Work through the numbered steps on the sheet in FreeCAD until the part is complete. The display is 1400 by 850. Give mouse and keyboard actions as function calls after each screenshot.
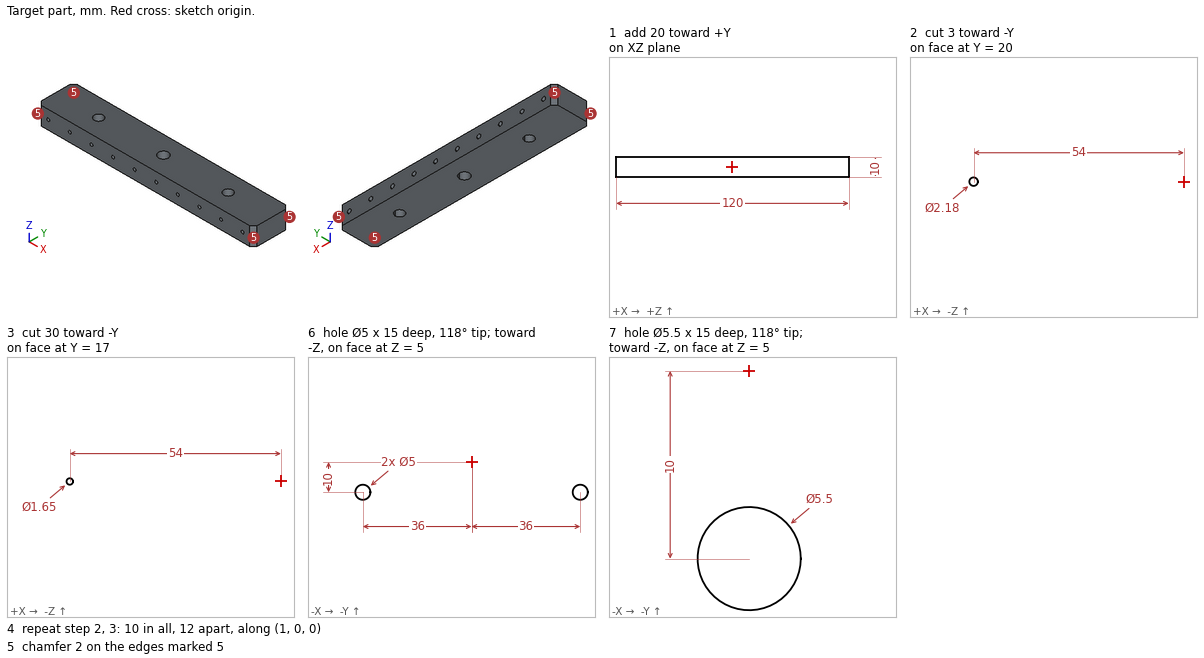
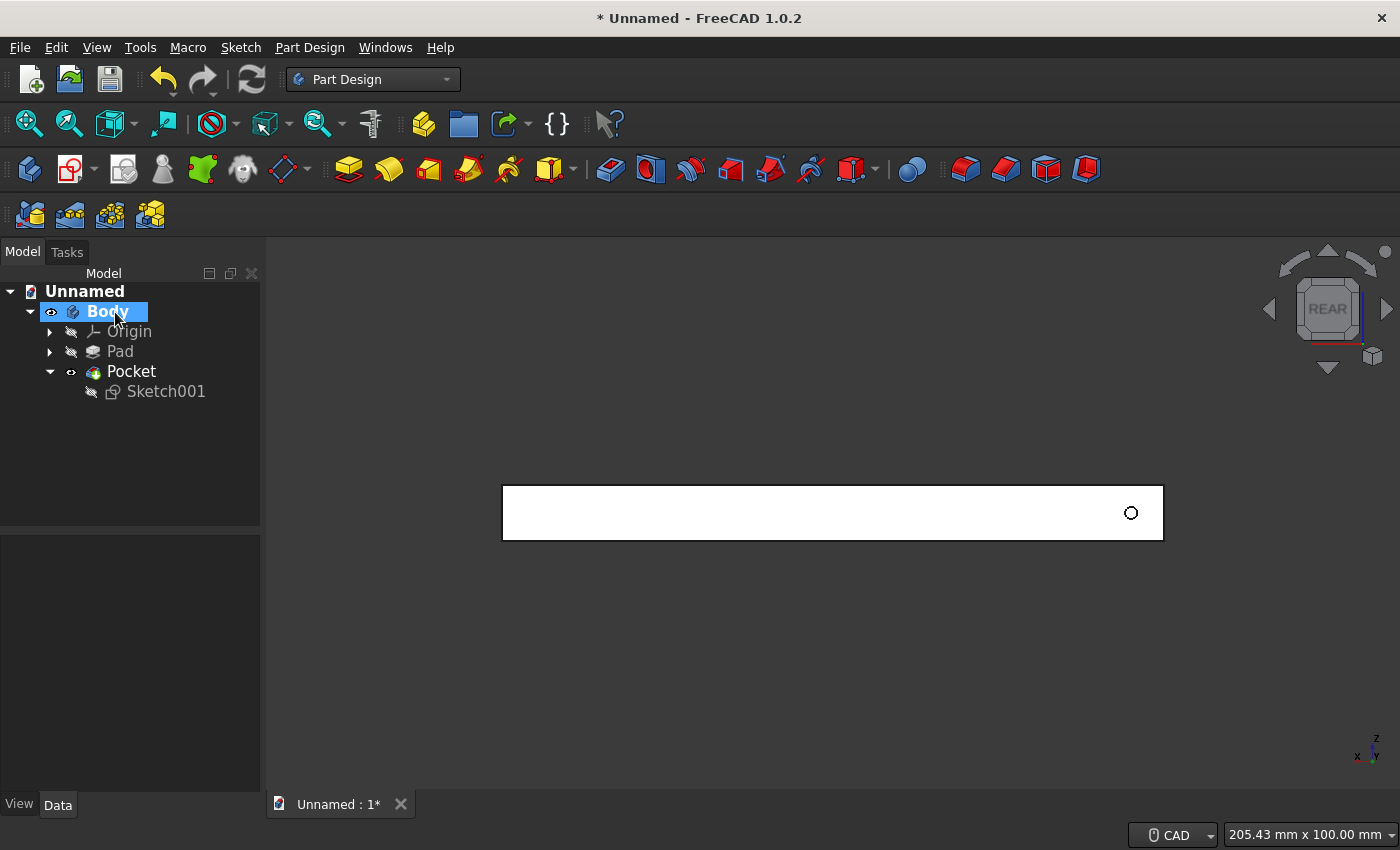
scroll(1131, 512, up, 4)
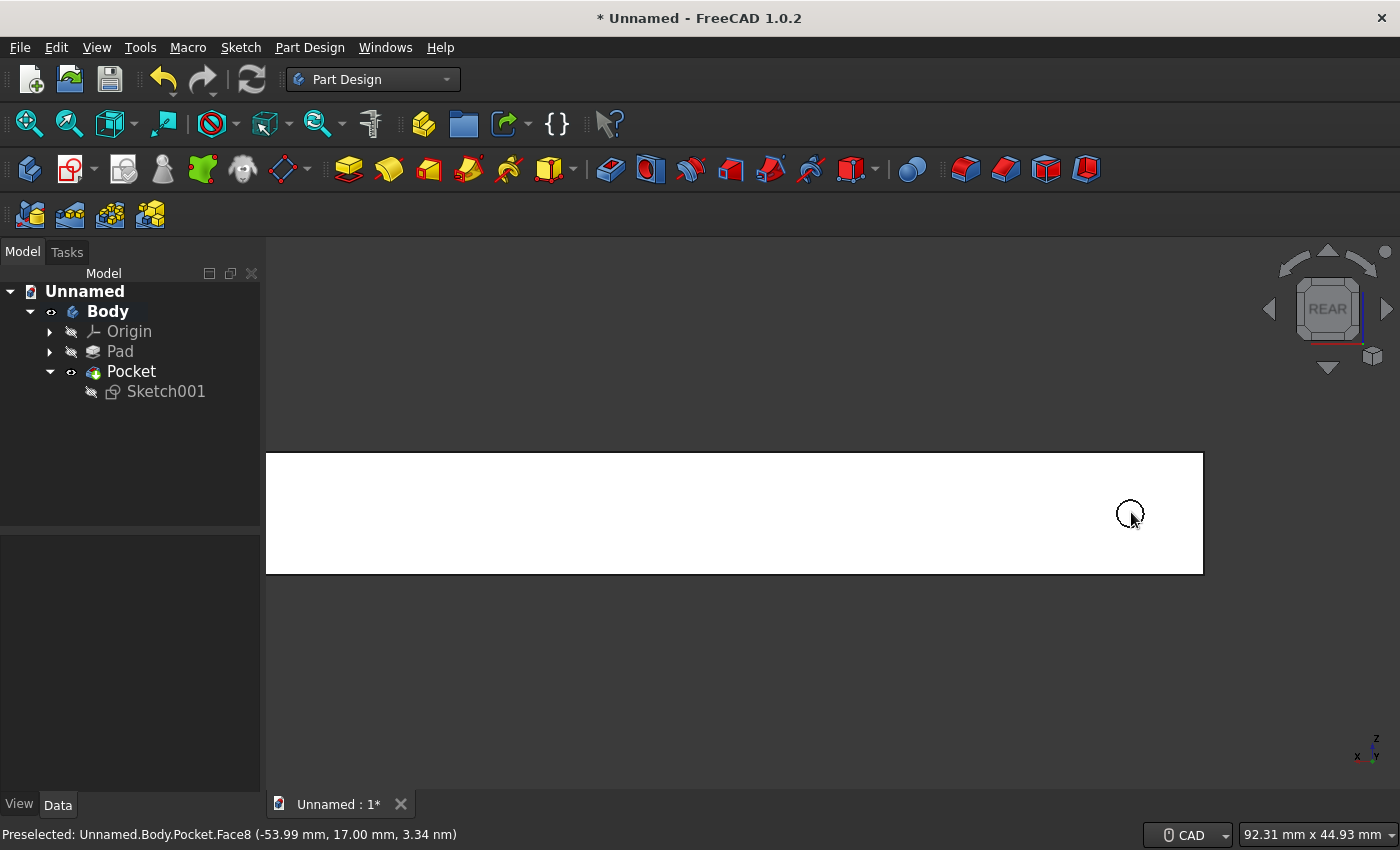
click(1130, 513)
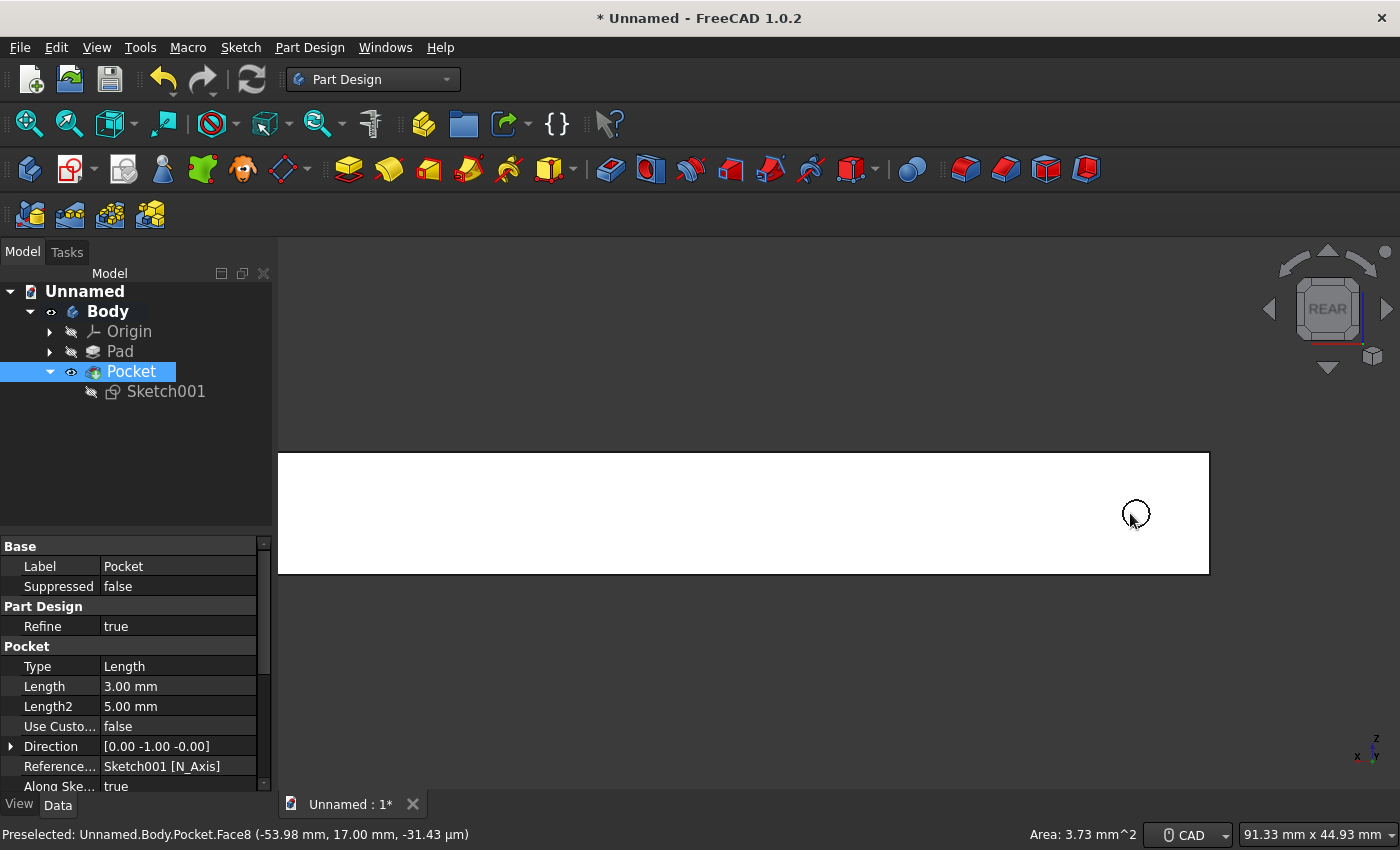
click(70, 170)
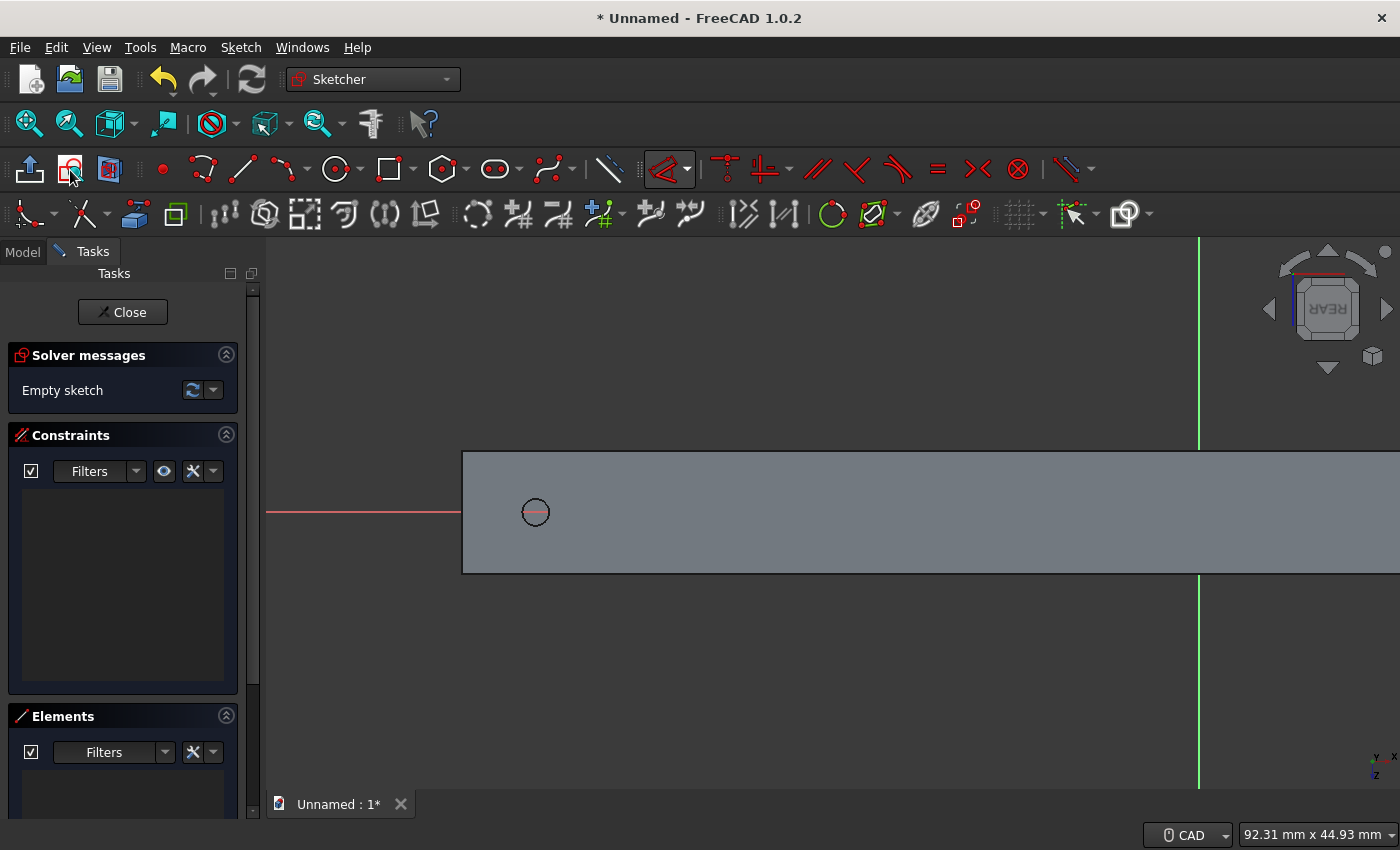
scroll(521, 512, up, 14)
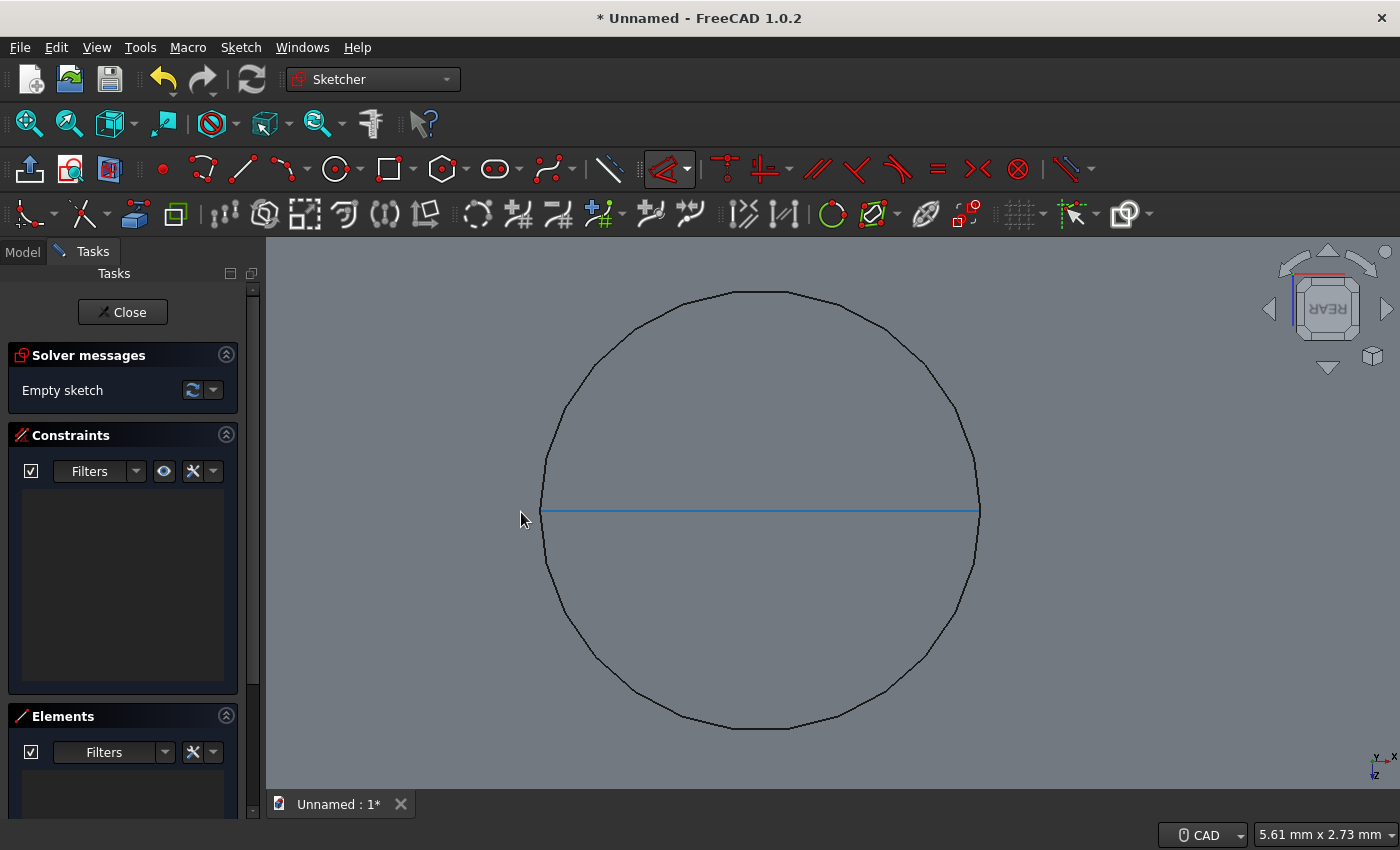
click(336, 170)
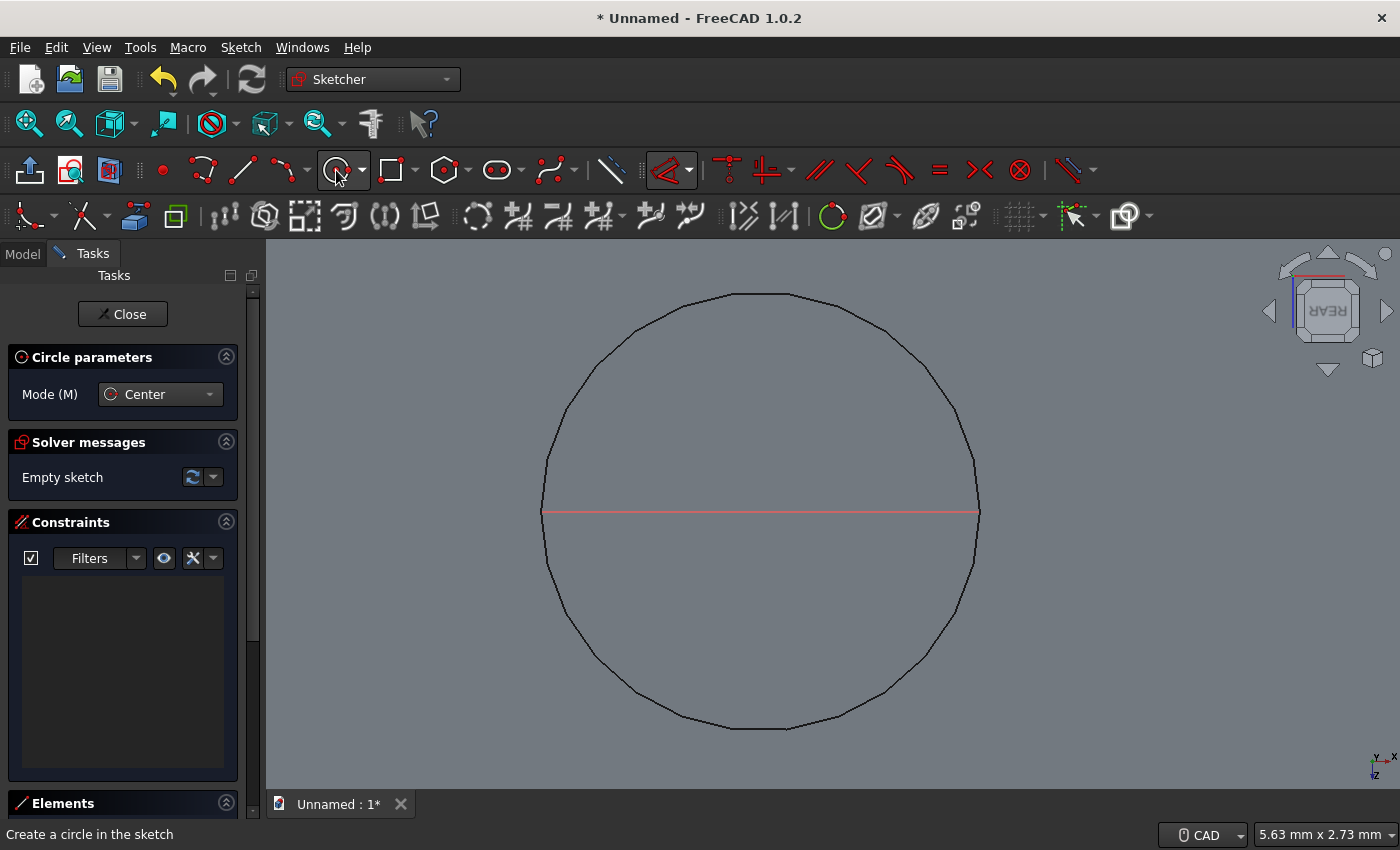
click(760, 512)
click(878, 394)
key(Escape)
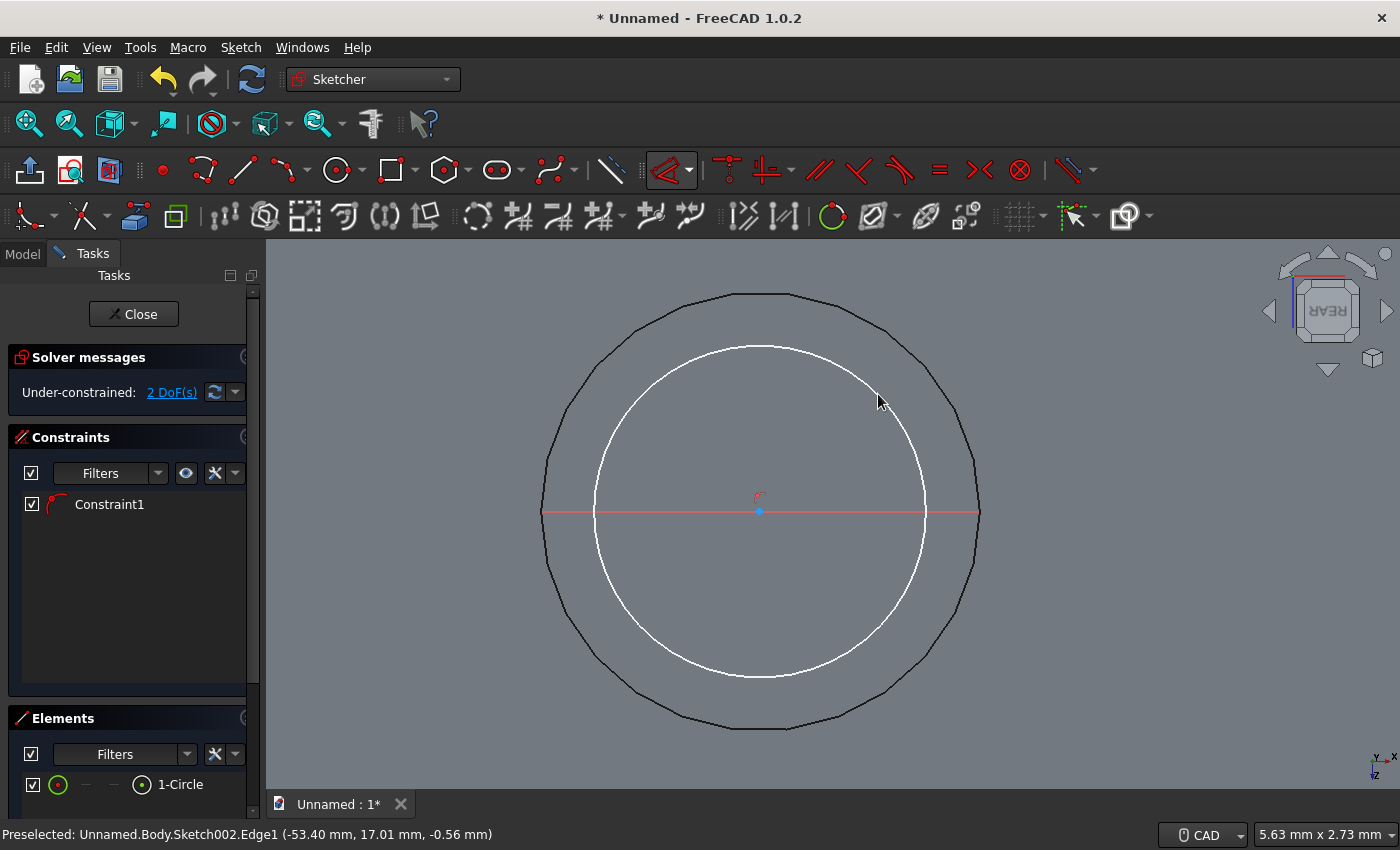
click(877, 394)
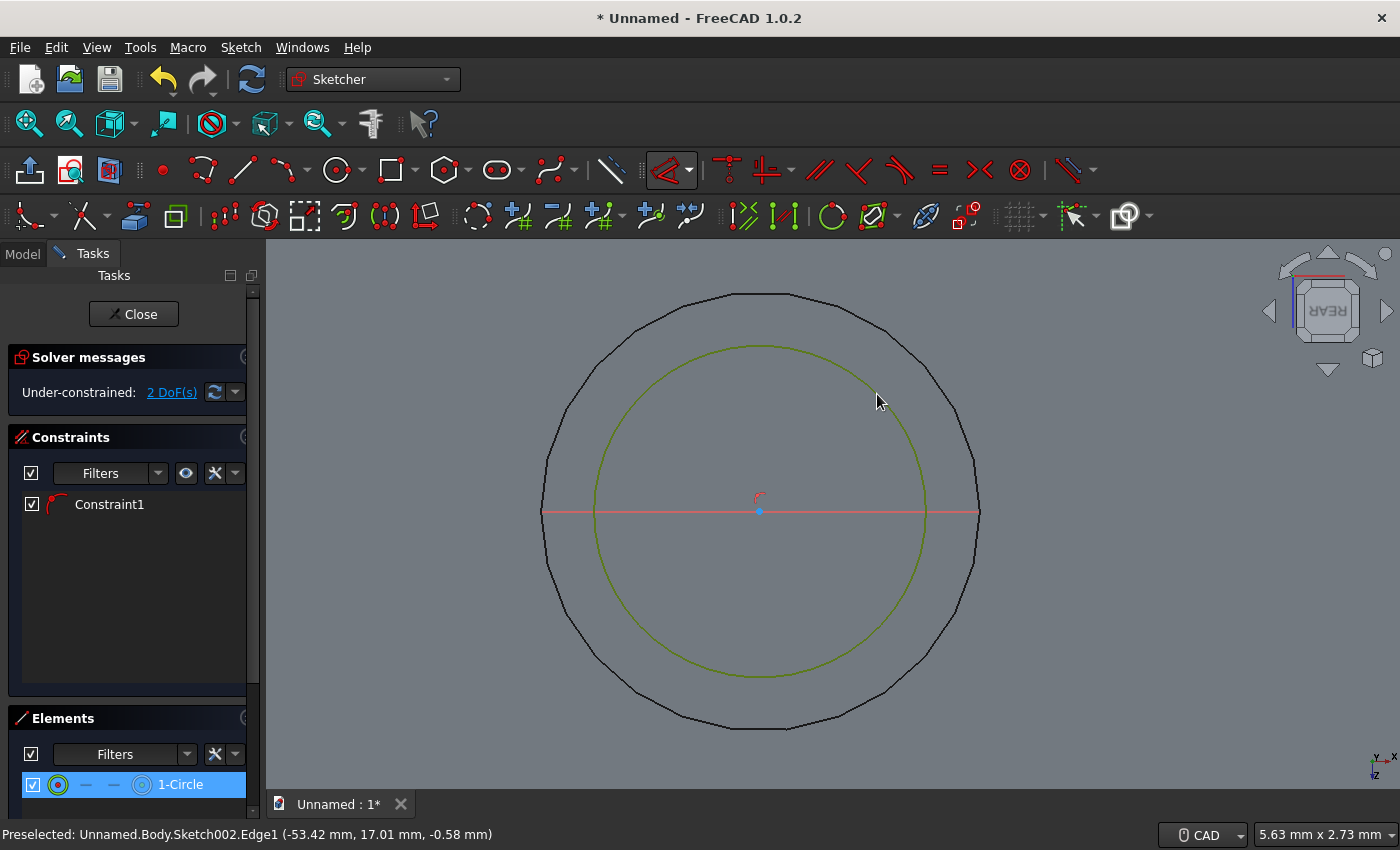
key(k)
key(o)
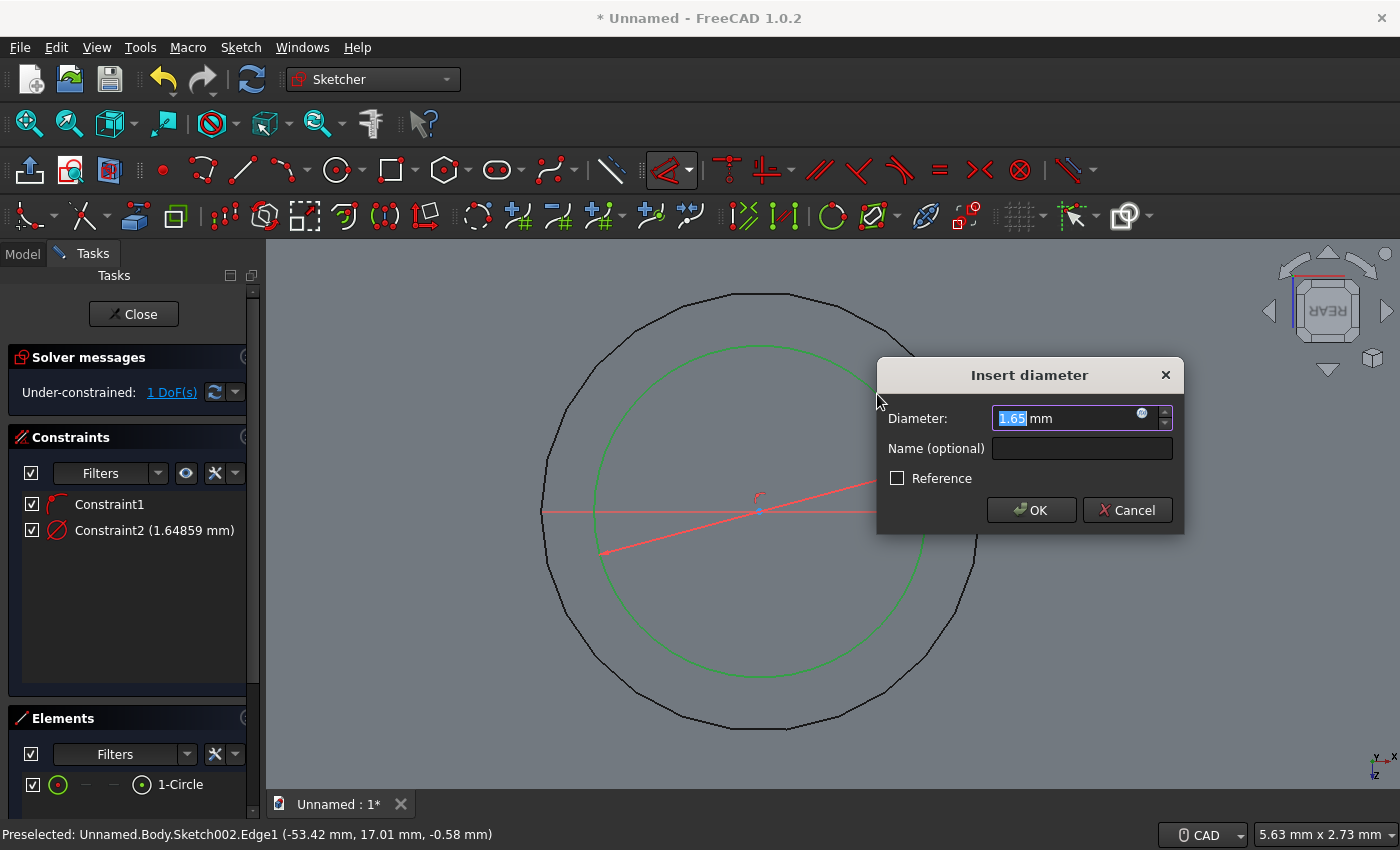
text(1.65)
key(Return)